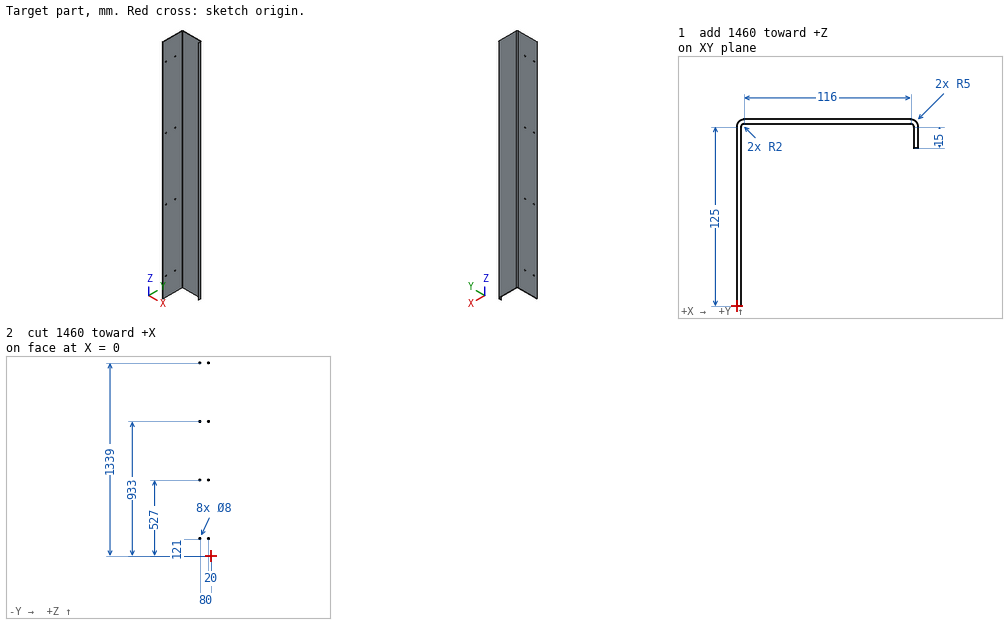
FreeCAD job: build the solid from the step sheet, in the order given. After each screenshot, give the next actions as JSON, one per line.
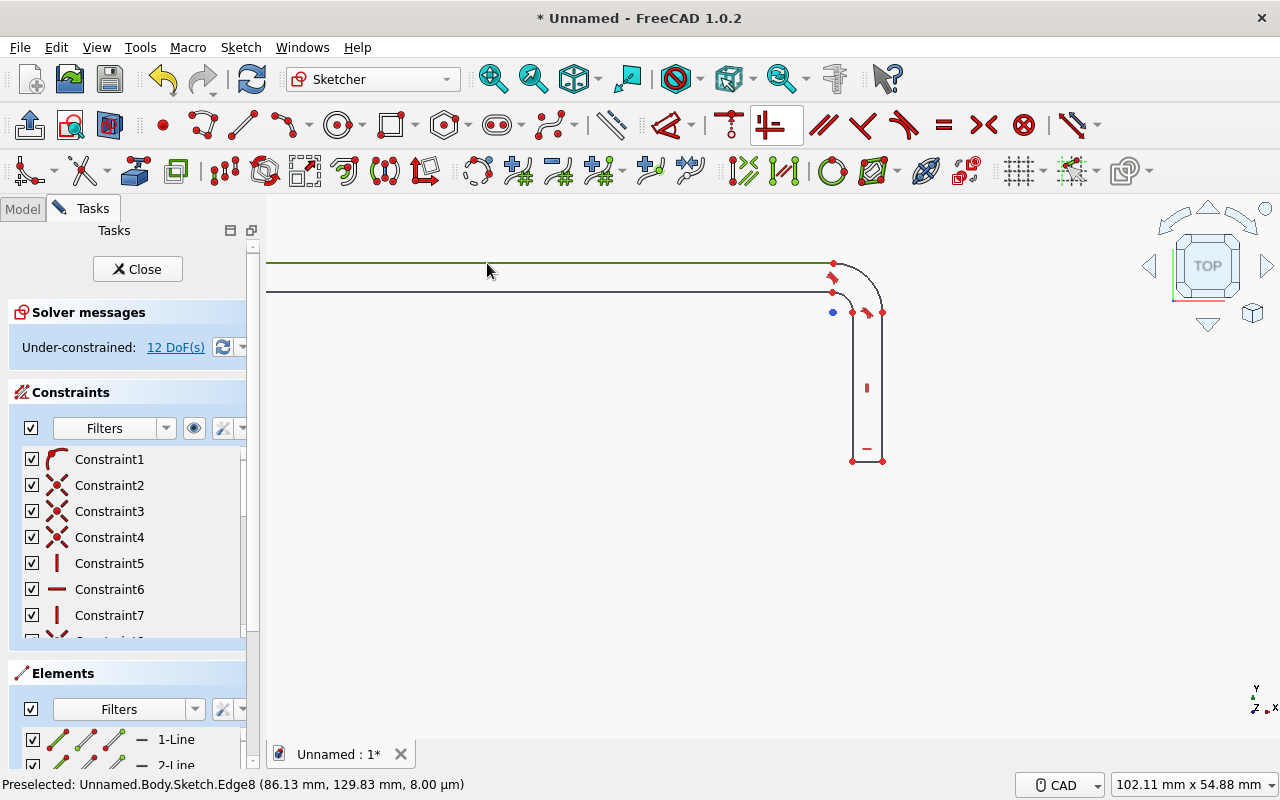
{"action": "scroll", "coordinate": [851, 322], "scroll_direction": "down", "scroll_amount": 7}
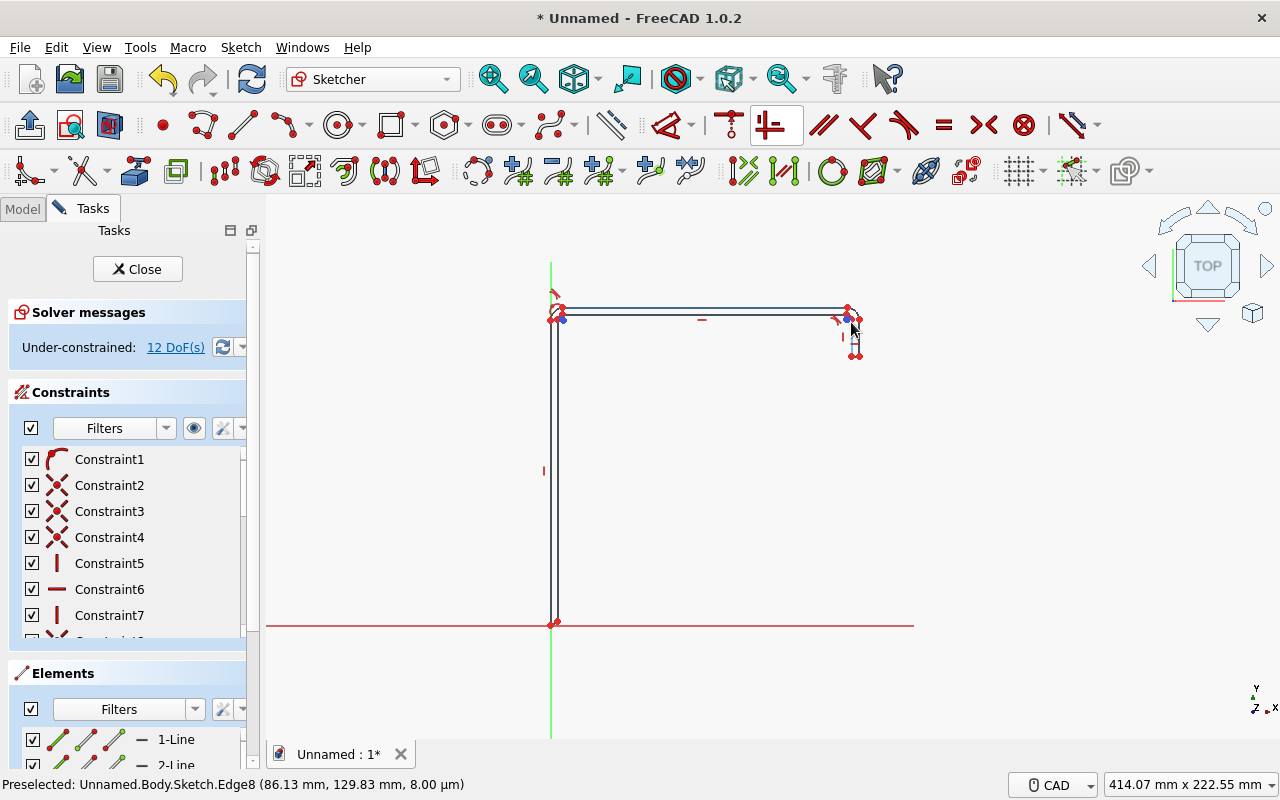
{"action": "scroll", "coordinate": [557, 309], "scroll_direction": "up", "scroll_amount": 5}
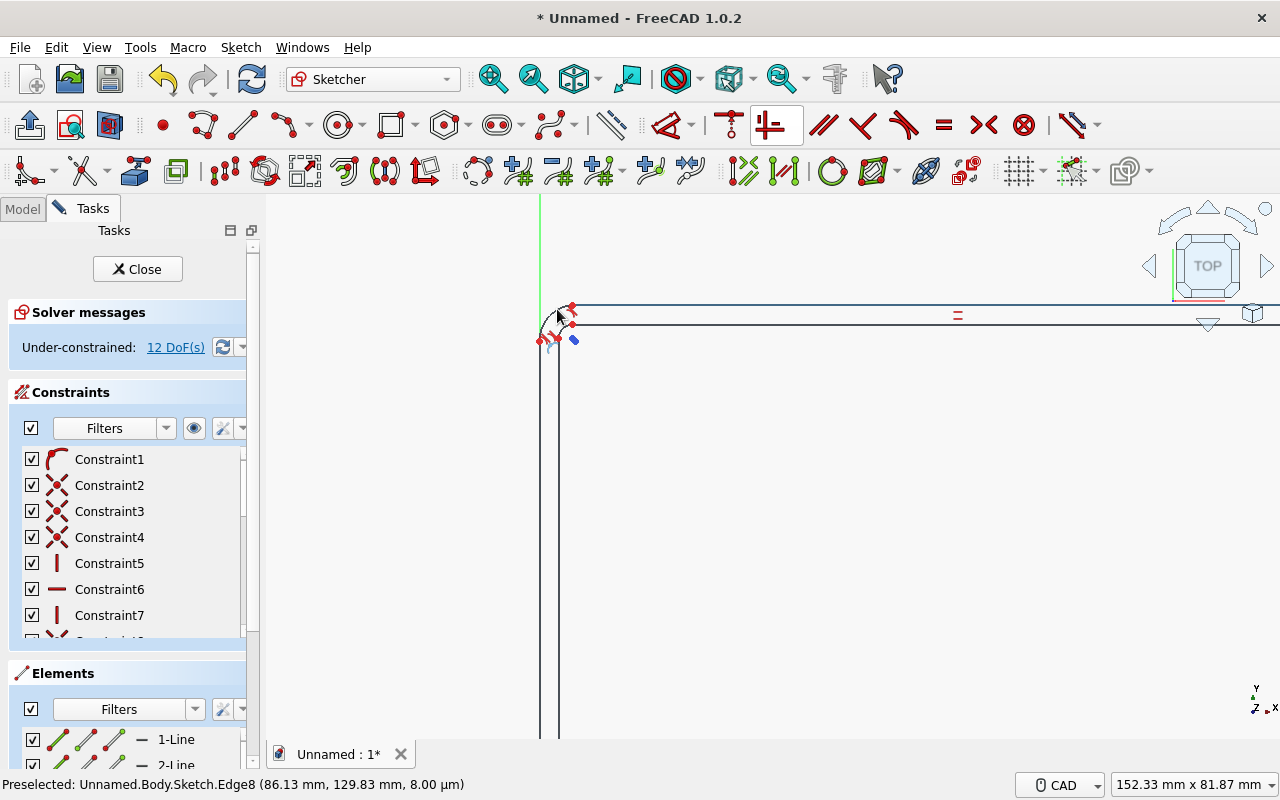
{"action": "left_click", "coordinate": [557, 310]}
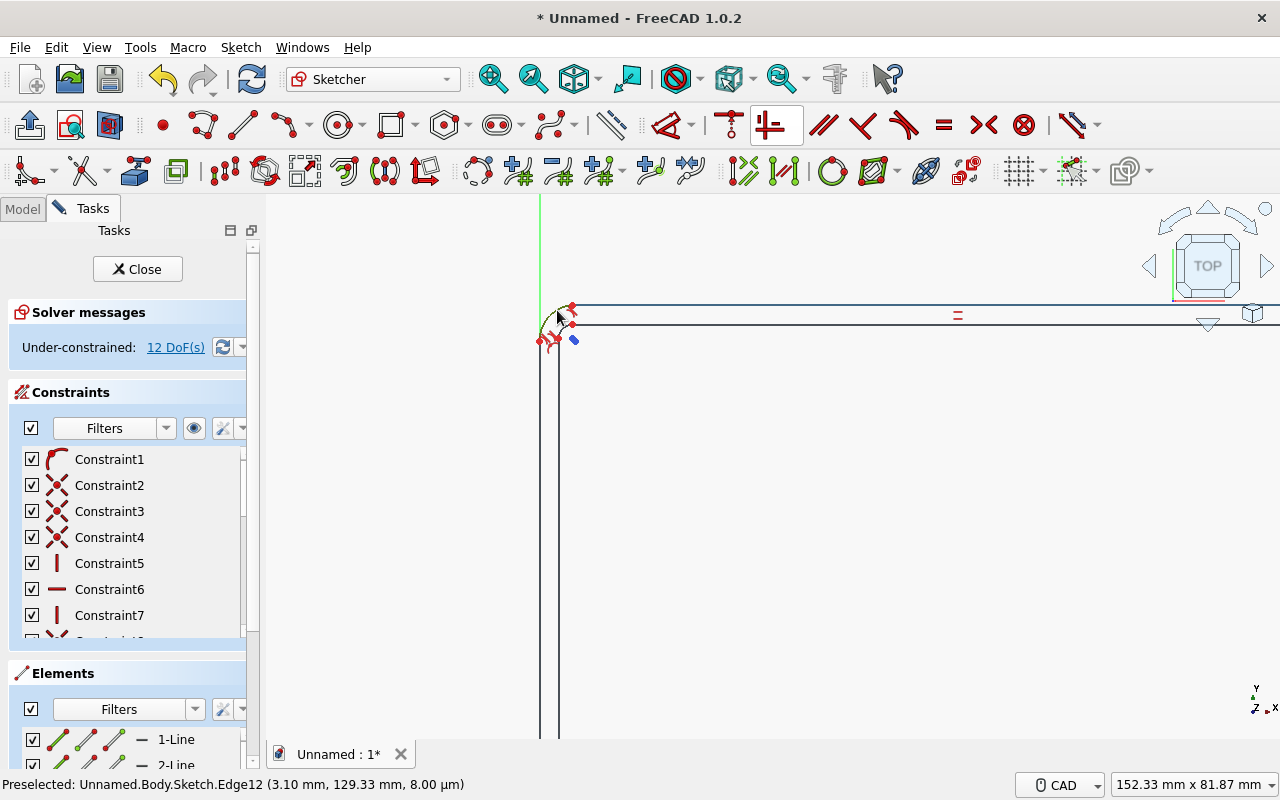
{"action": "left_click", "coordinate": [904, 126]}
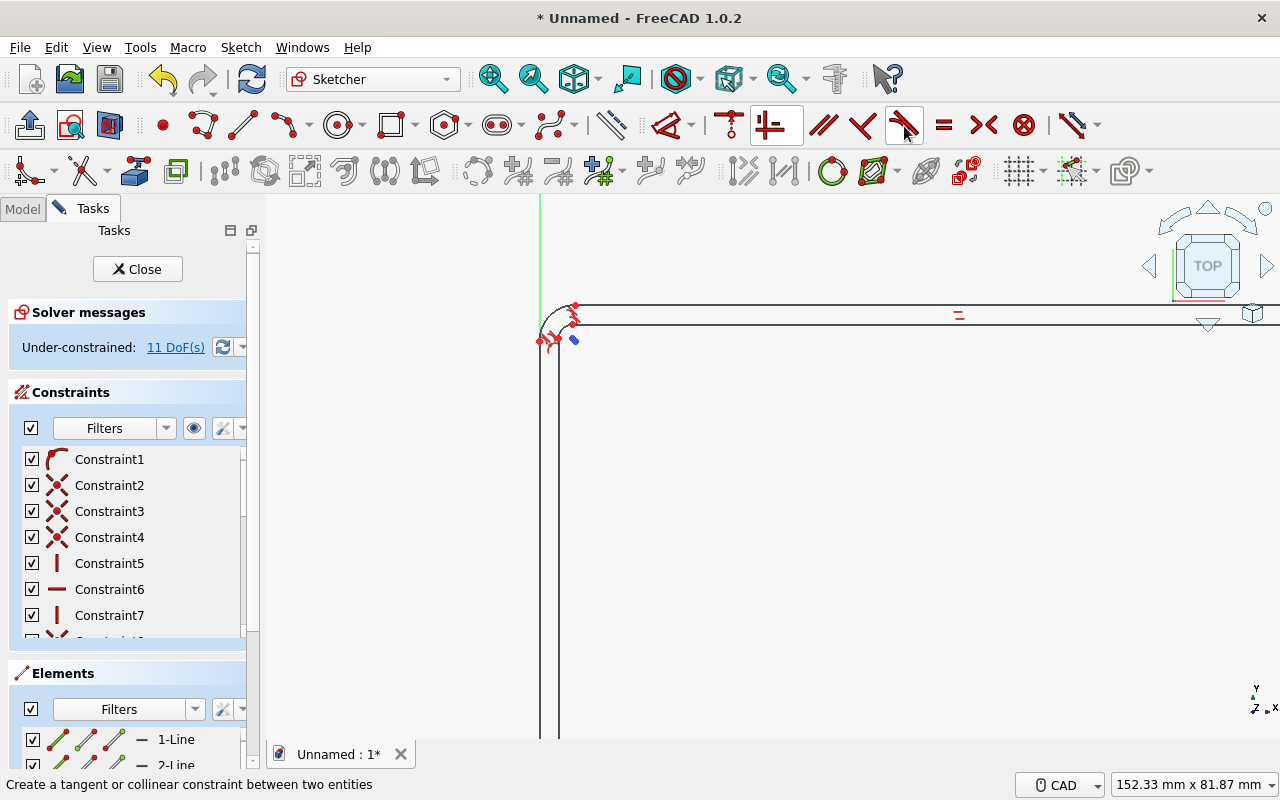
{"action": "scroll", "coordinate": [556, 309], "scroll_direction": "down", "scroll_amount": 5}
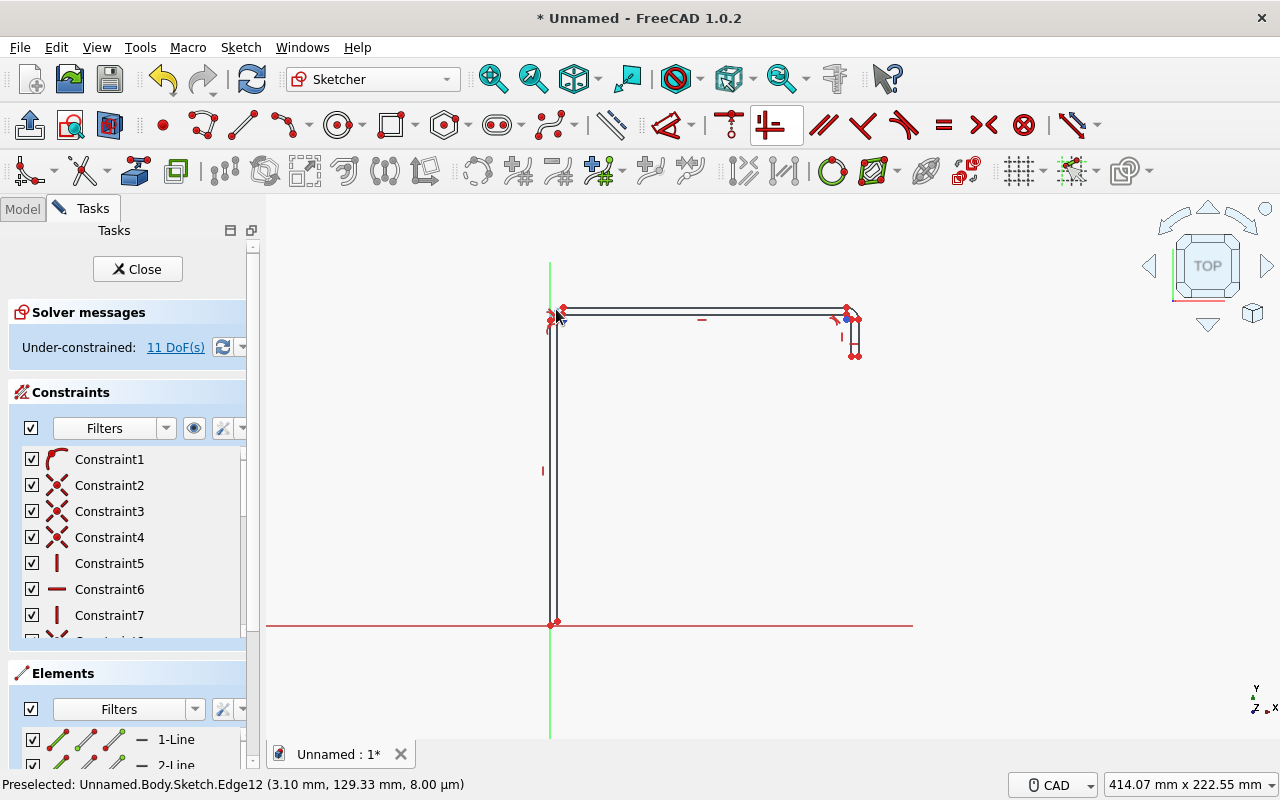
{"action": "scroll", "coordinate": [555, 623], "scroll_direction": "up", "scroll_amount": 9}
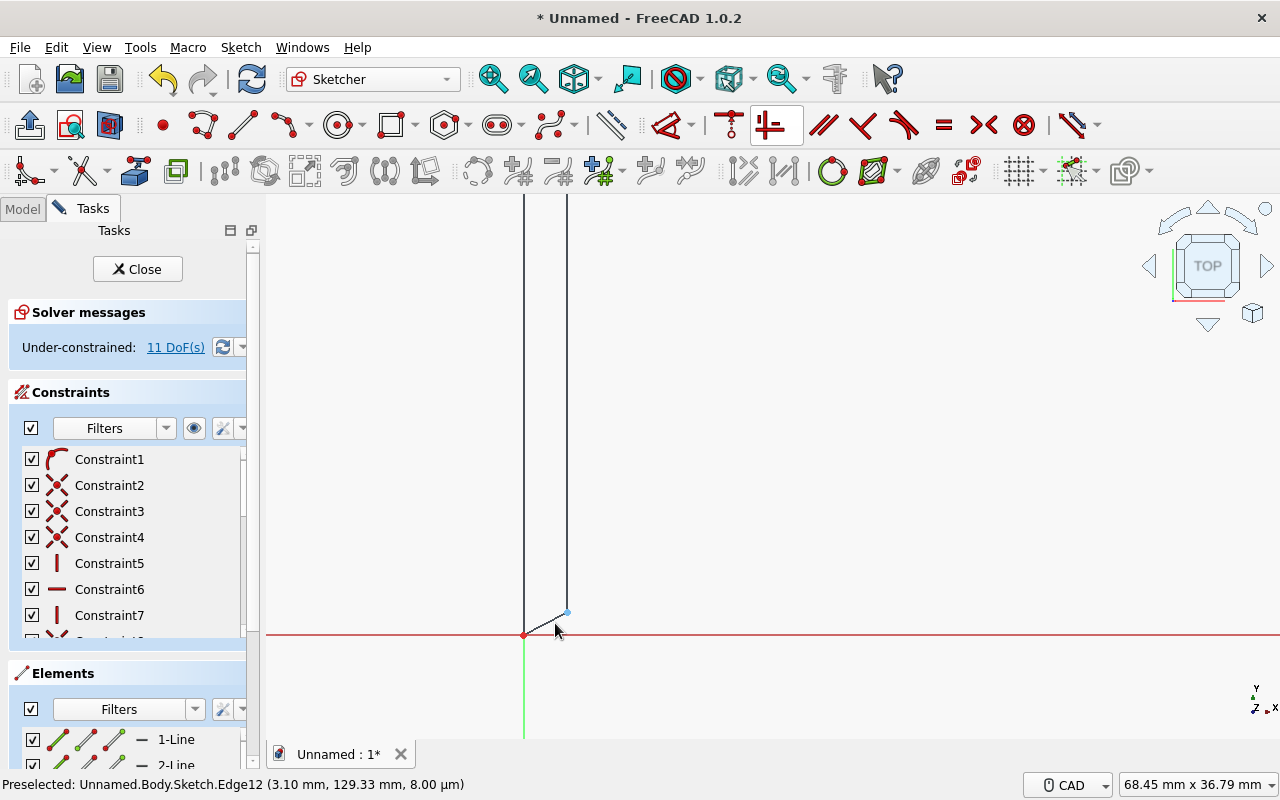
{"action": "left_click", "coordinate": [554, 619]}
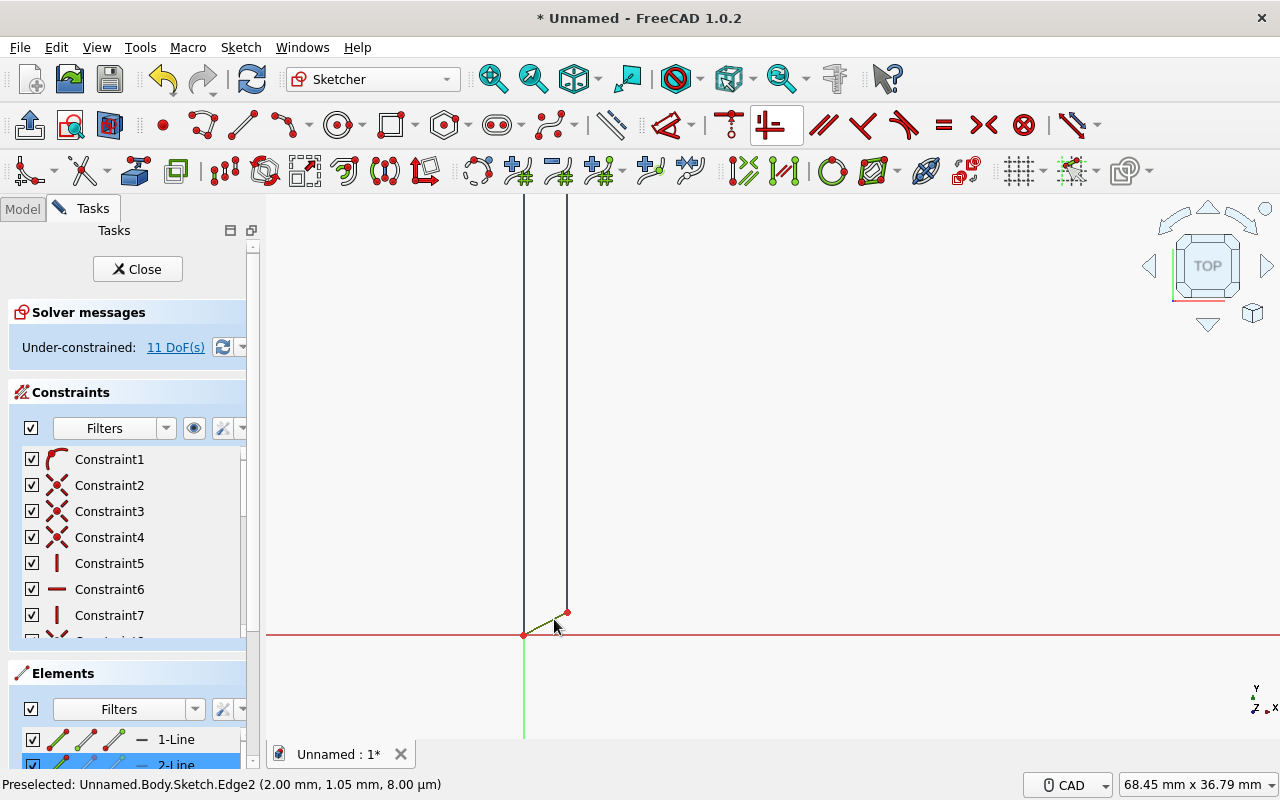
{"action": "key", "text": "h"}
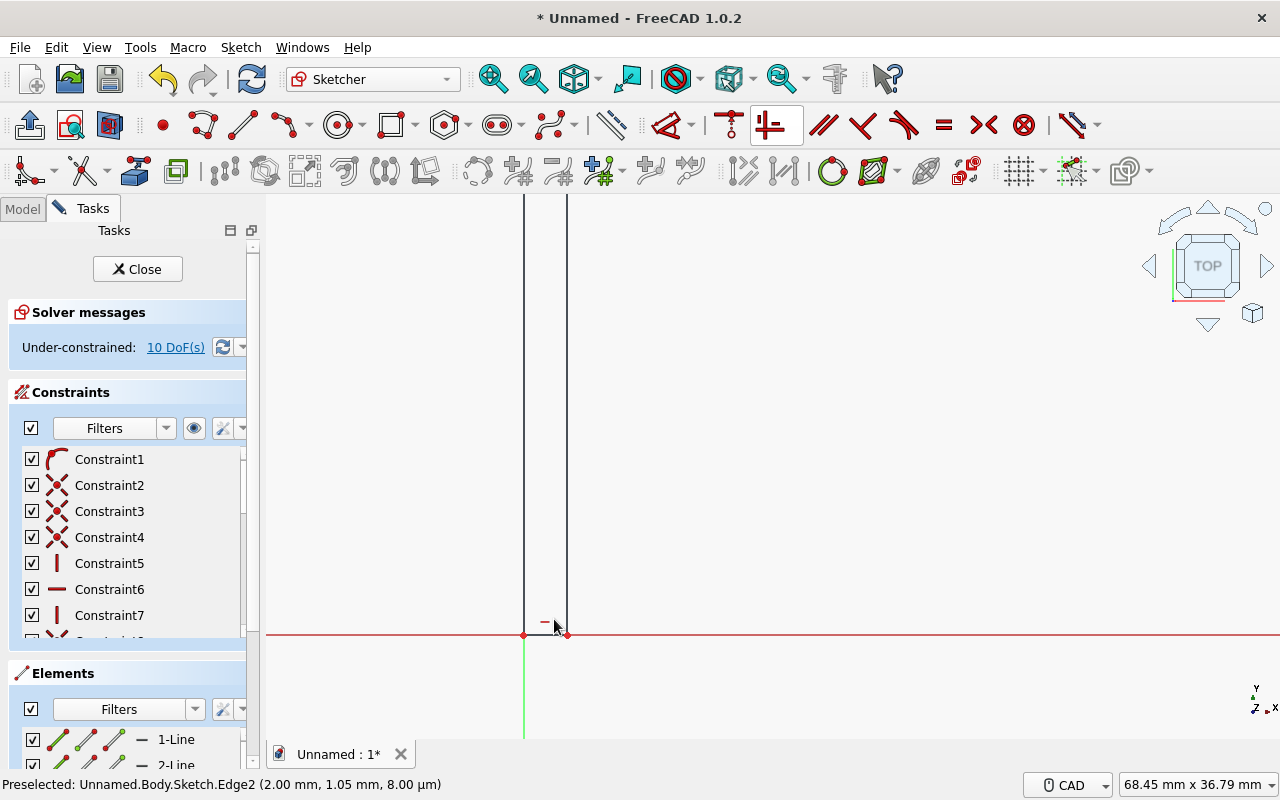
{"action": "scroll", "coordinate": [555, 624], "scroll_direction": "down", "scroll_amount": 9}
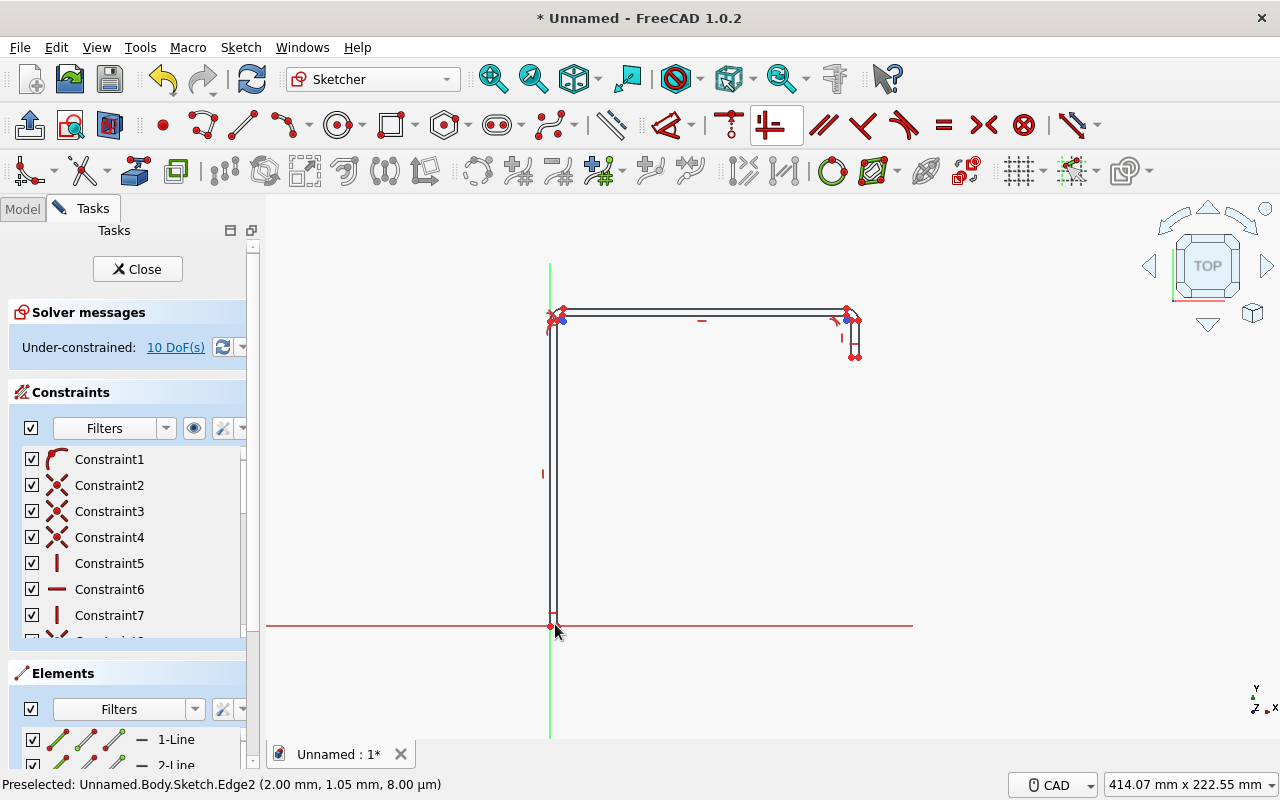
{"action": "scroll", "coordinate": [851, 318], "scroll_direction": "up", "scroll_amount": 9}